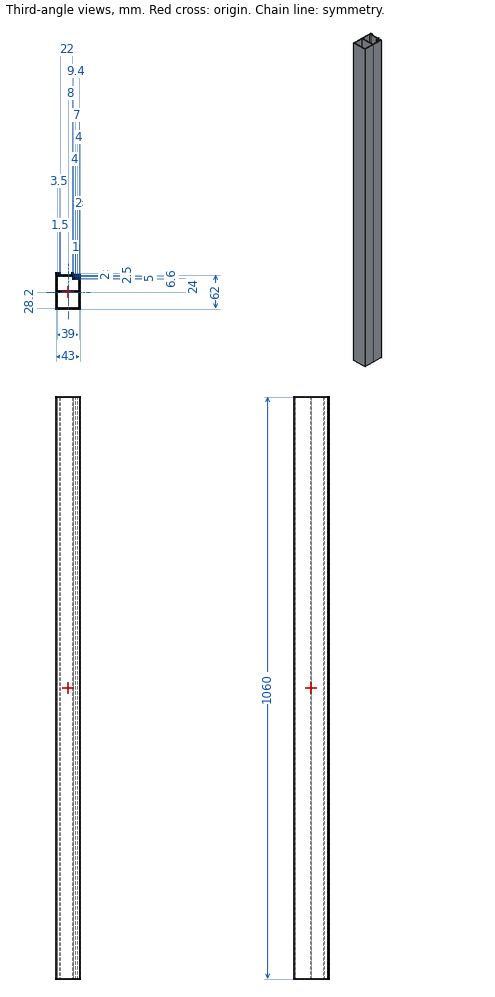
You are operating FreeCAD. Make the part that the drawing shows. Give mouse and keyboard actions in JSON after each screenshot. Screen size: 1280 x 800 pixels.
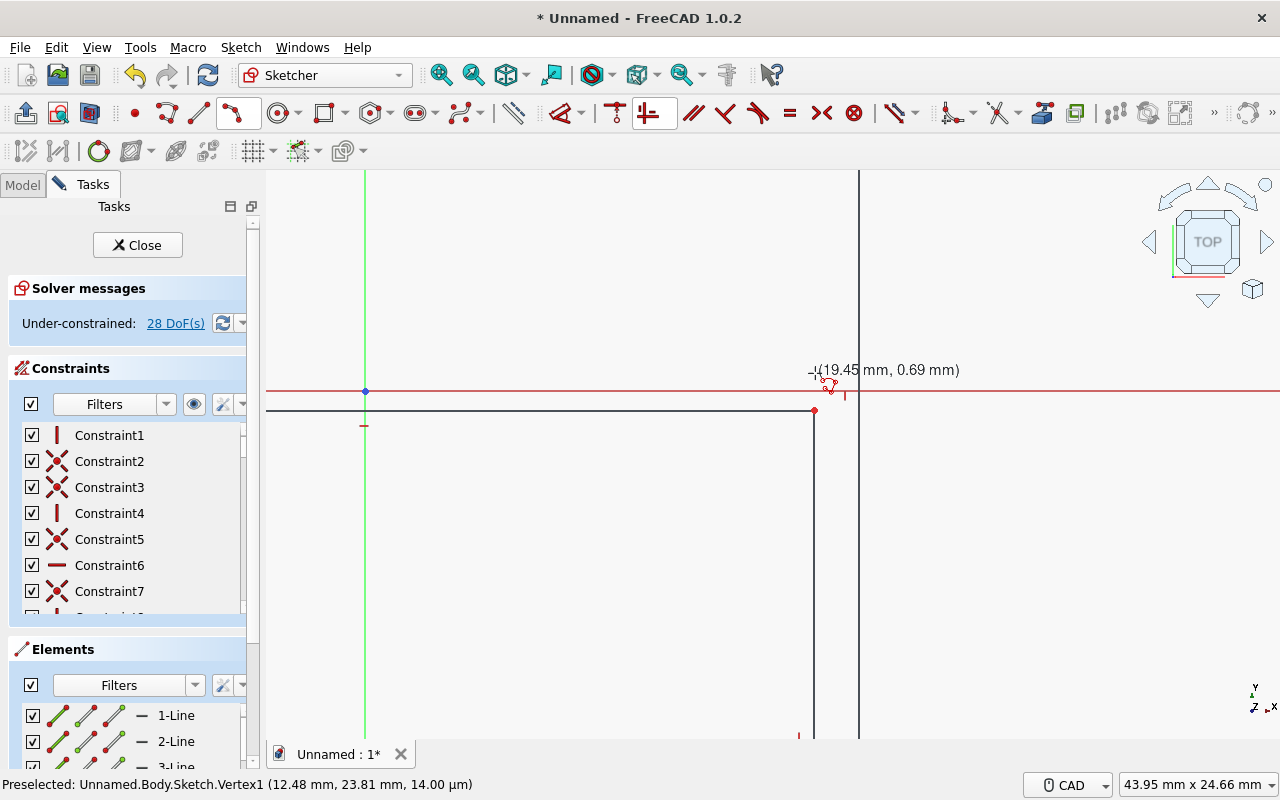
{"action": "left_click", "coordinate": [815, 373]}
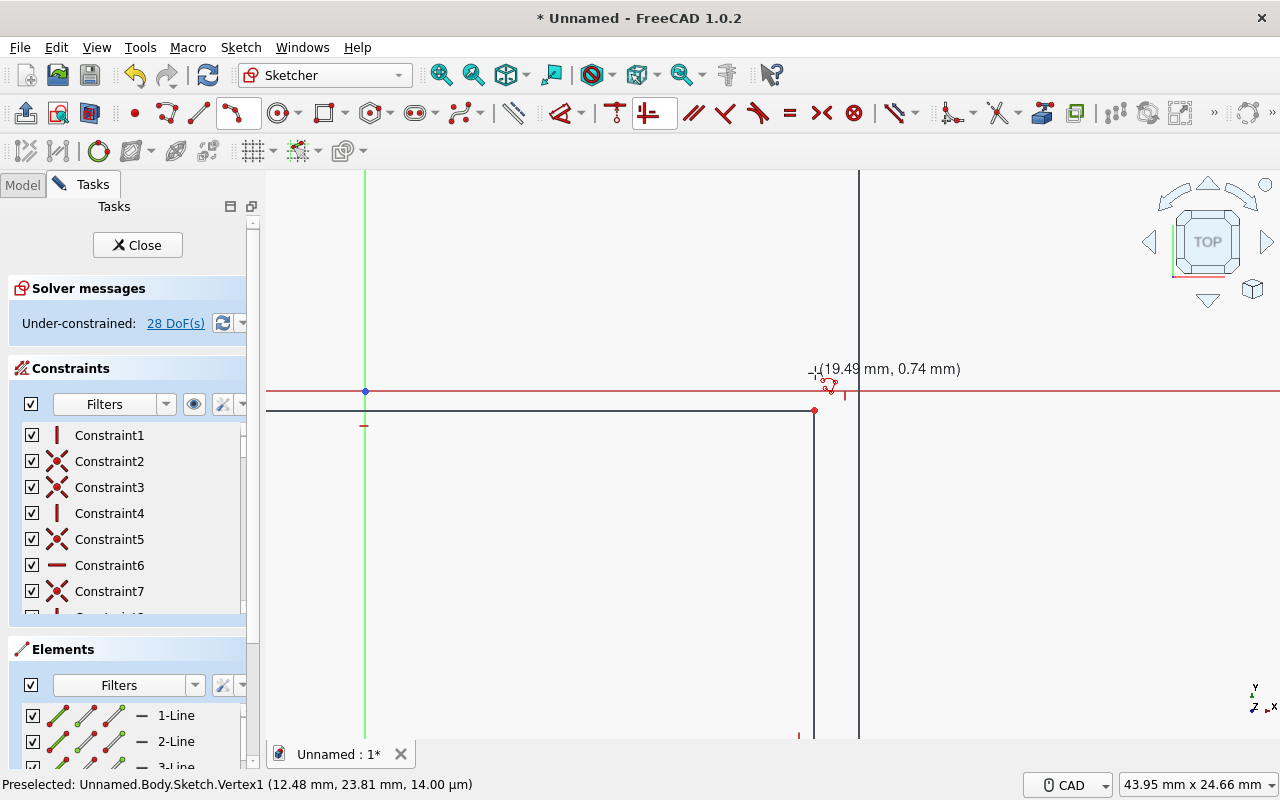
{"action": "scroll", "coordinate": [816, 485], "scroll_direction": "down", "scroll_amount": 7}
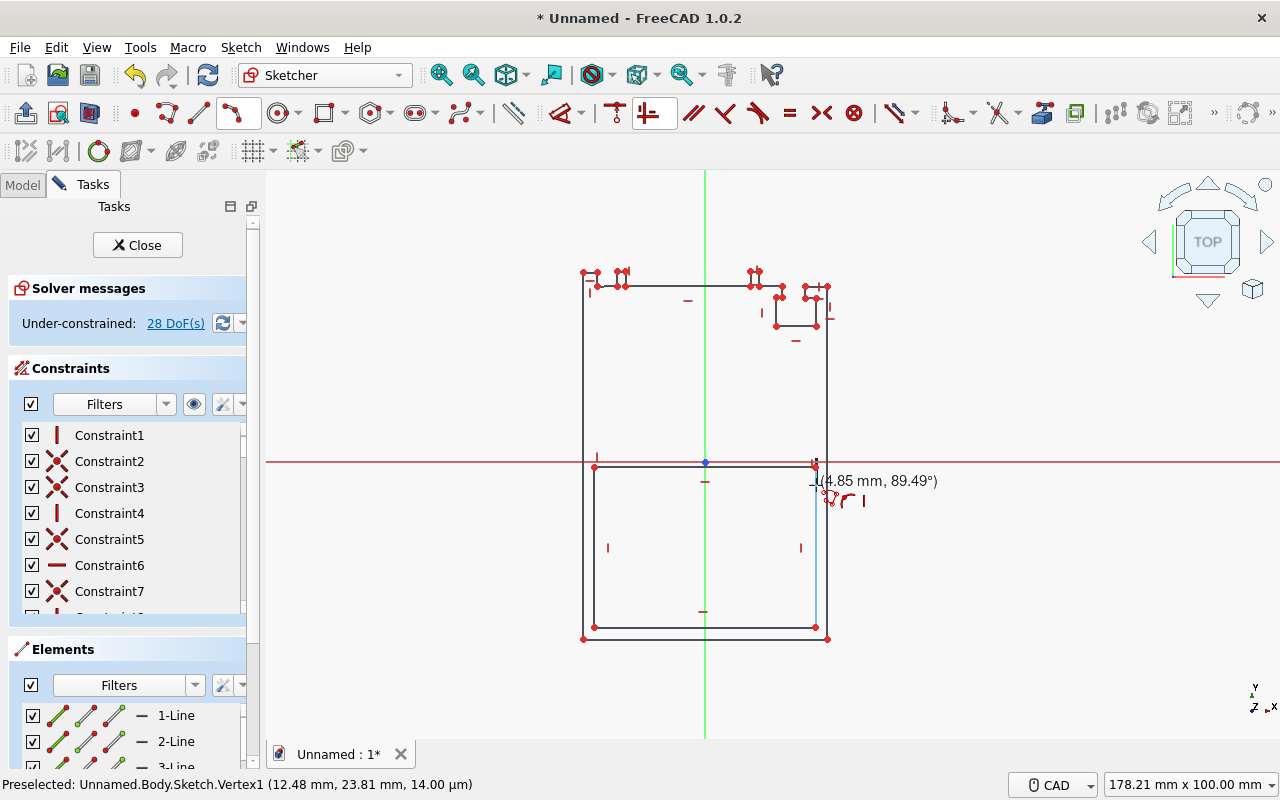
{"action": "scroll", "coordinate": [594, 458], "scroll_direction": "up", "scroll_amount": 7}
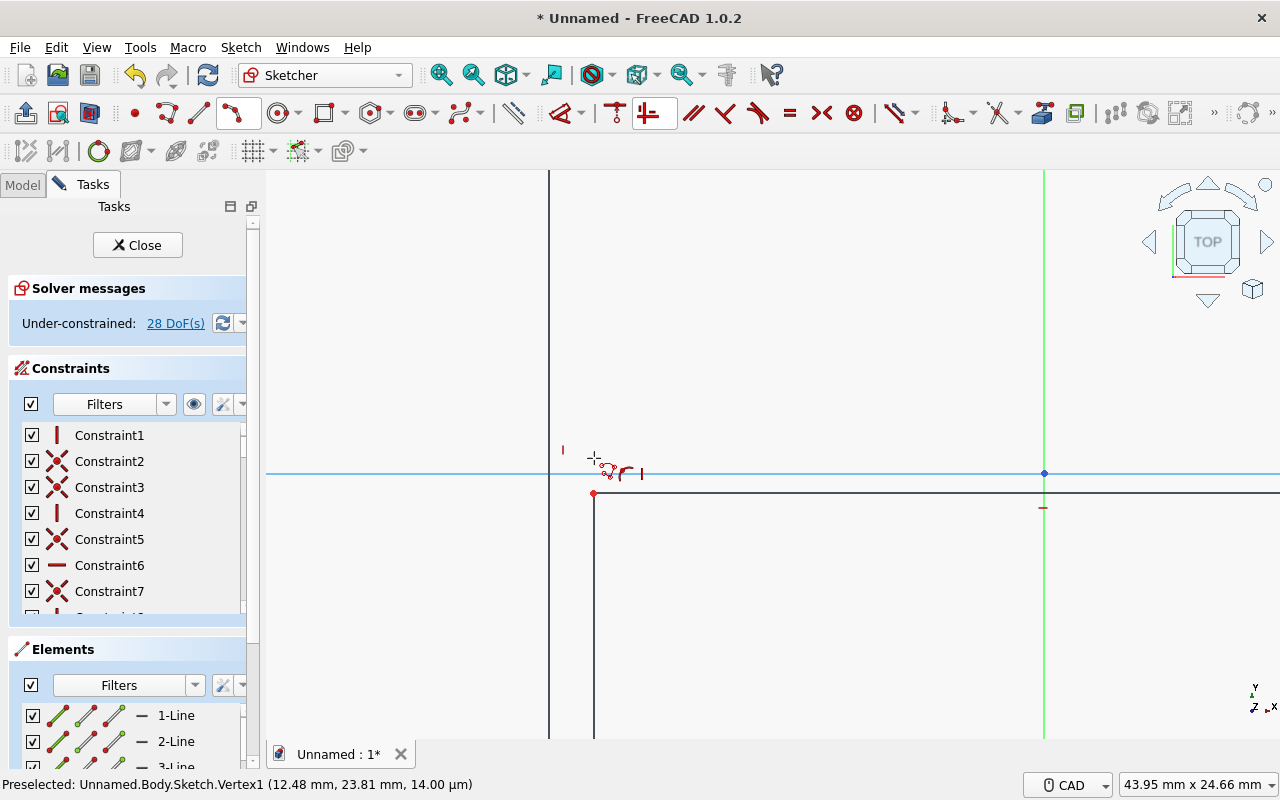
{"action": "left_click", "coordinate": [594, 456]}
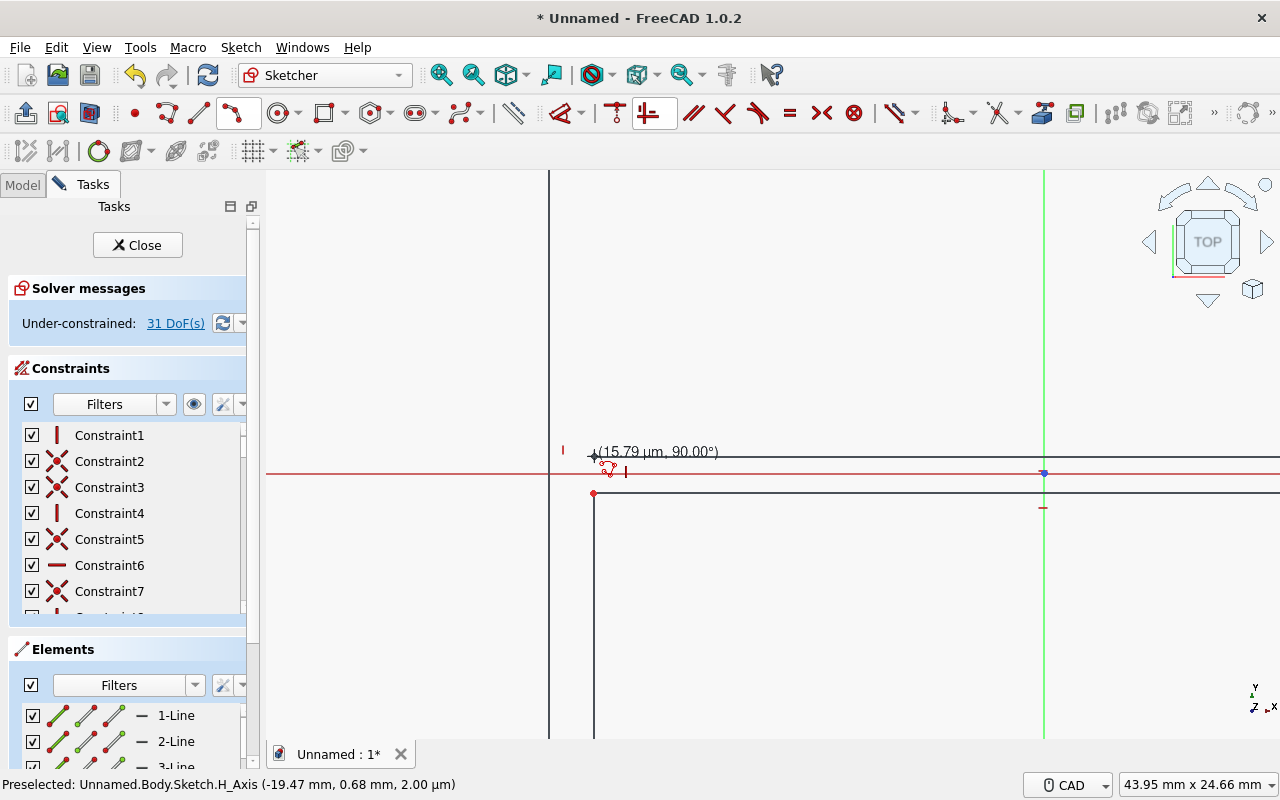
{"action": "scroll", "coordinate": [593, 458], "scroll_direction": "down", "scroll_amount": 7}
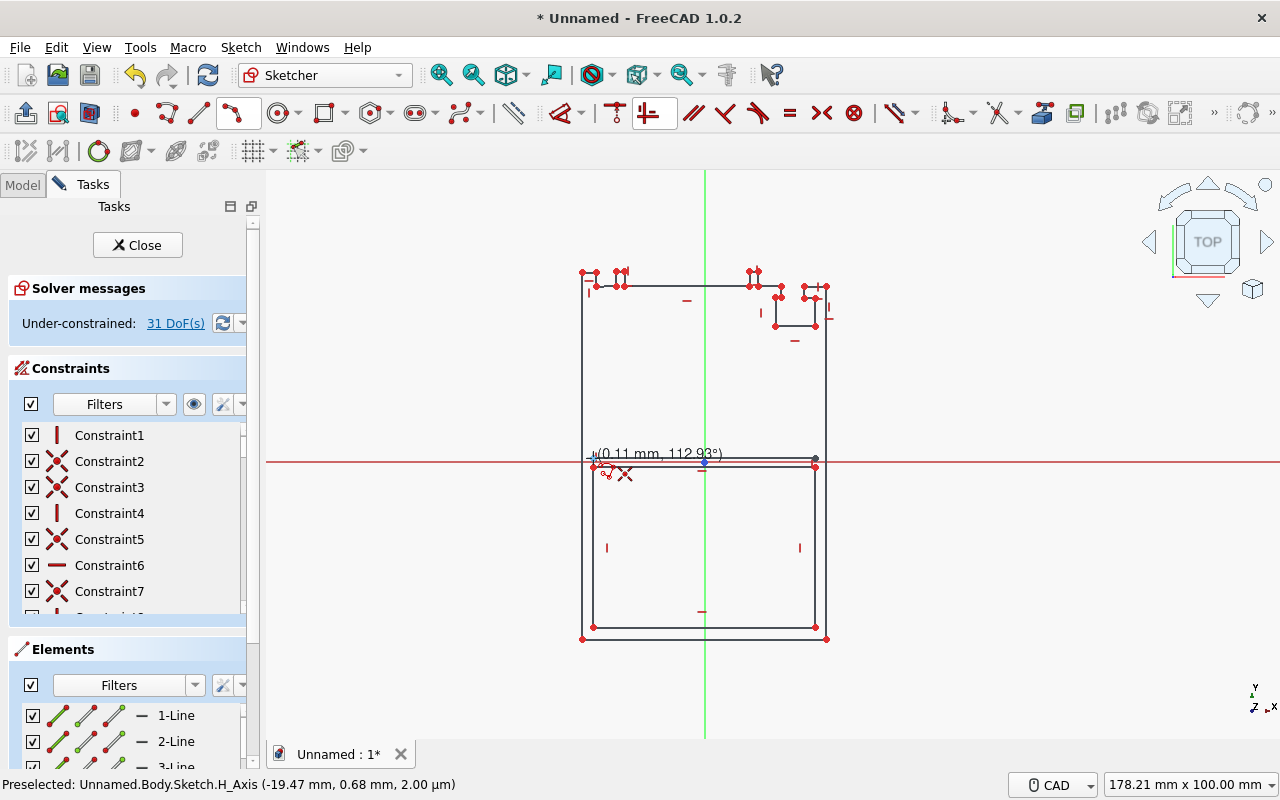
{"action": "scroll", "coordinate": [594, 297], "scroll_direction": "up", "scroll_amount": 2}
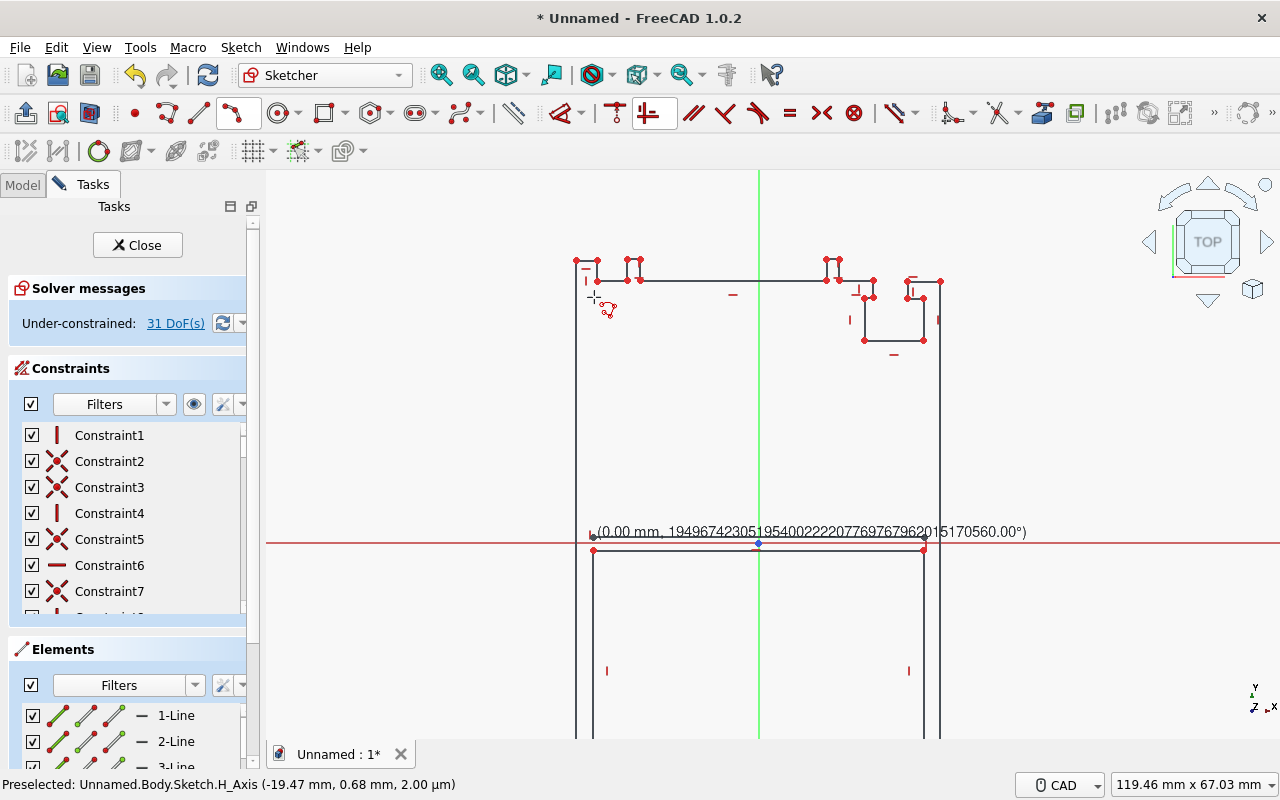
{"action": "left_click", "coordinate": [593, 297]}
{"action": "left_click", "coordinate": [844, 297]}
{"action": "left_click", "coordinate": [844, 353]}
{"action": "left_click", "coordinate": [924, 353]}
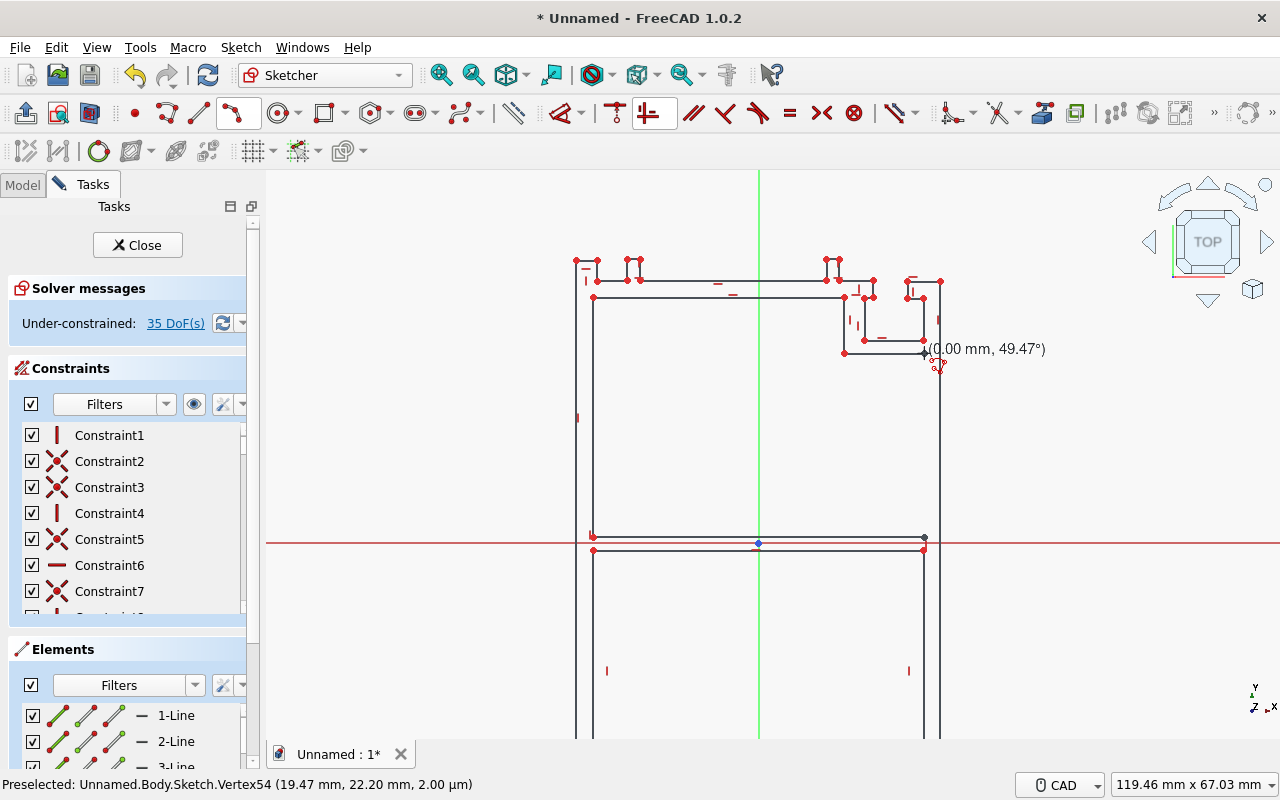
{"action": "scroll", "coordinate": [924, 537], "scroll_direction": "up", "scroll_amount": 5}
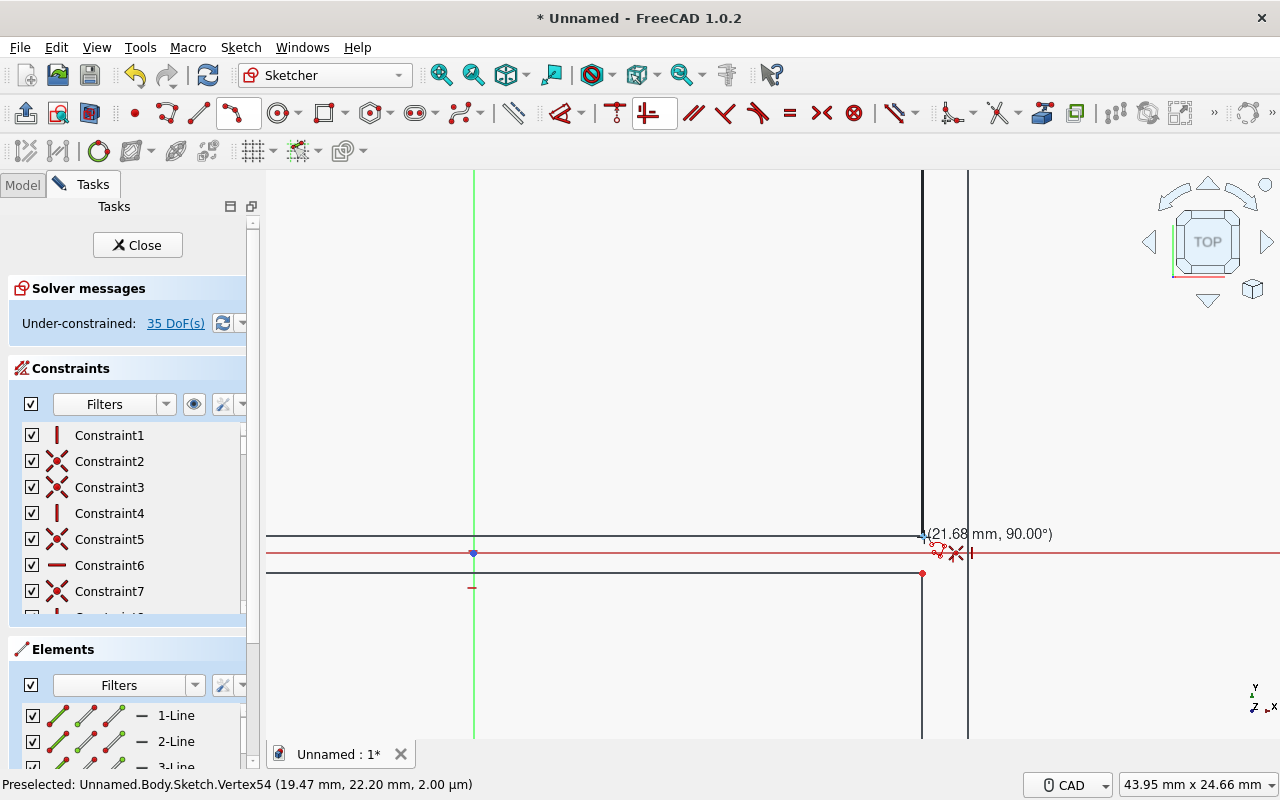
{"action": "left_click", "coordinate": [923, 536]}
{"action": "key", "text": "Escape"}
{"action": "key", "text": "Escape"}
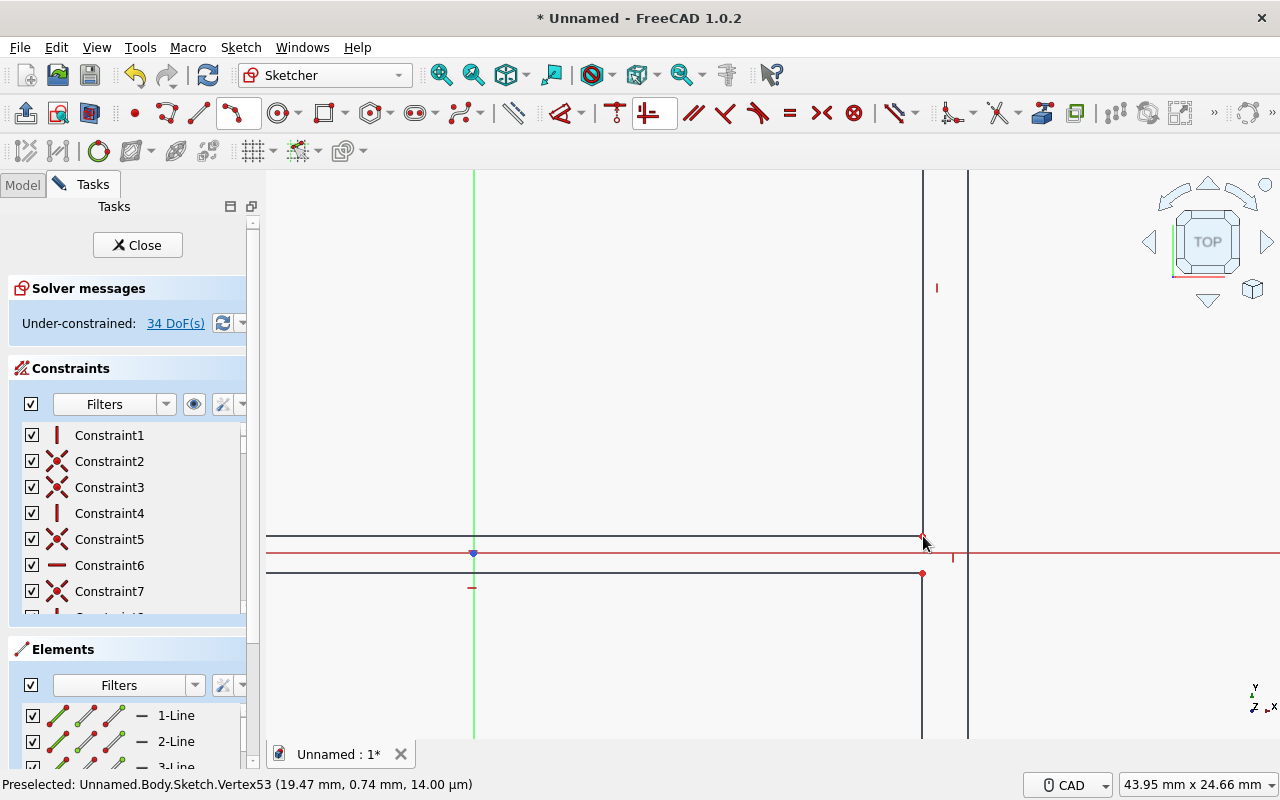
{"action": "scroll", "coordinate": [780, 432], "scroll_direction": "down", "scroll_amount": 7}